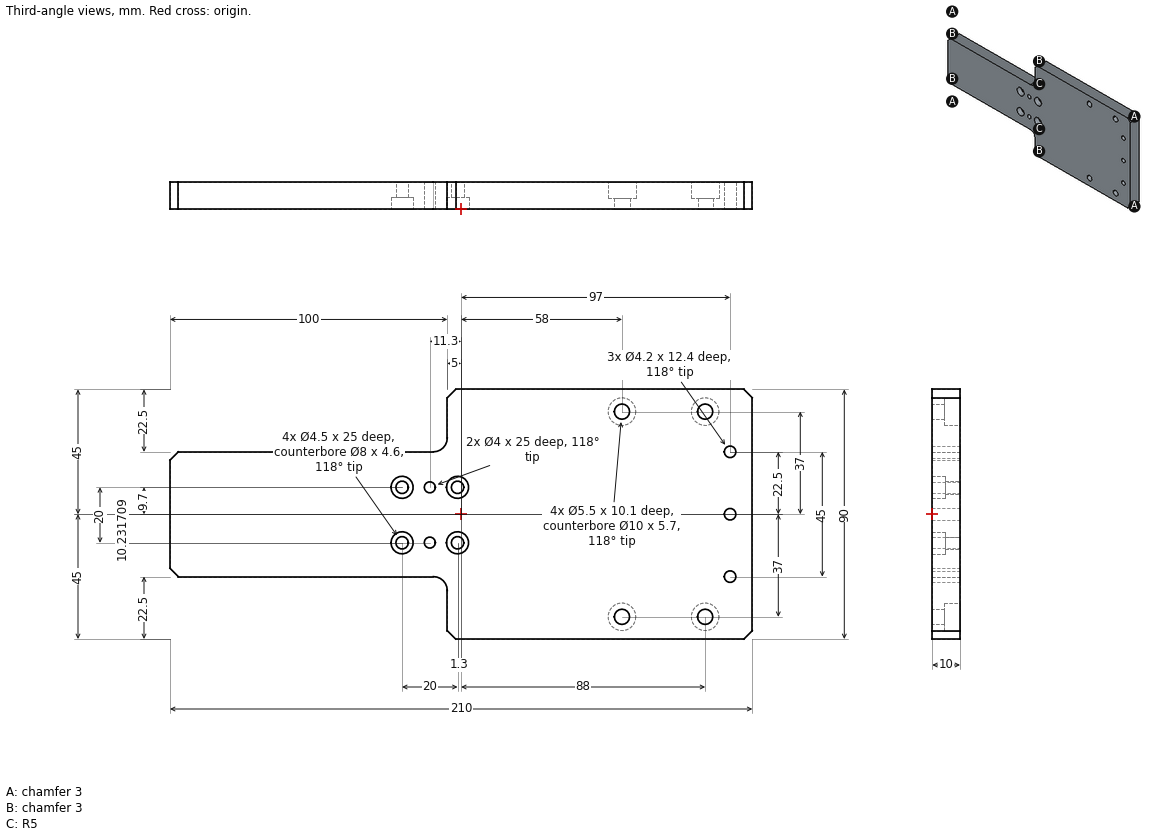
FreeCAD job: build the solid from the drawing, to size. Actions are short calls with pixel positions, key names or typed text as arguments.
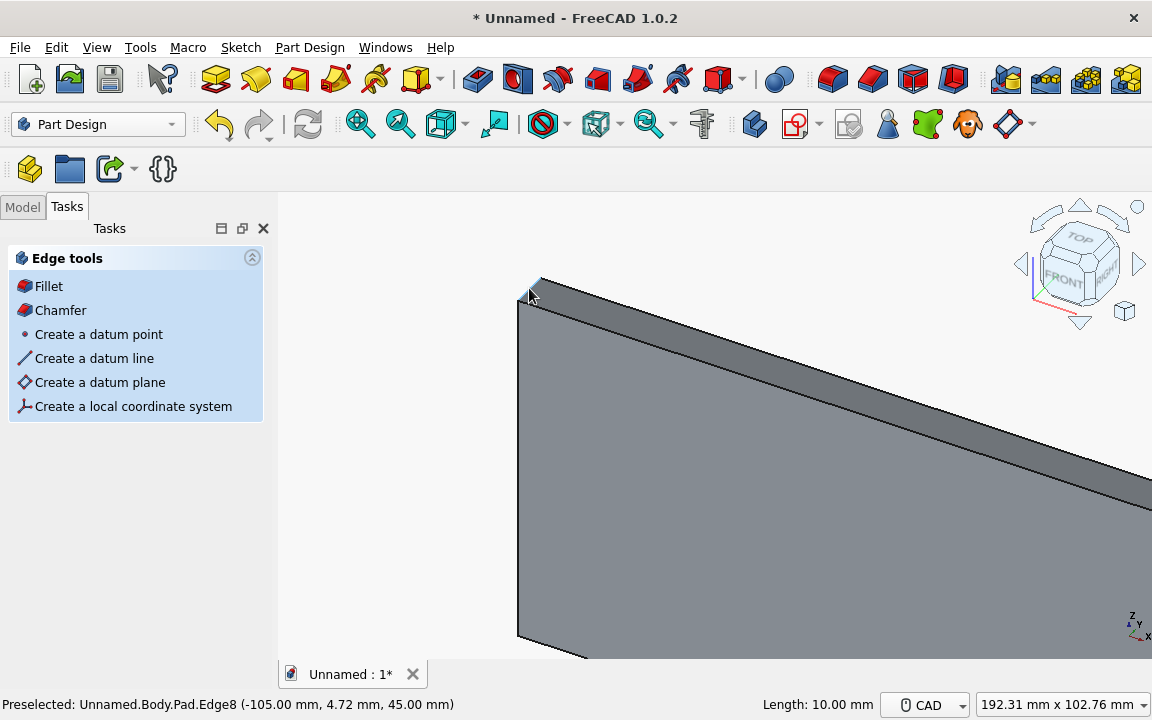
click(362, 124)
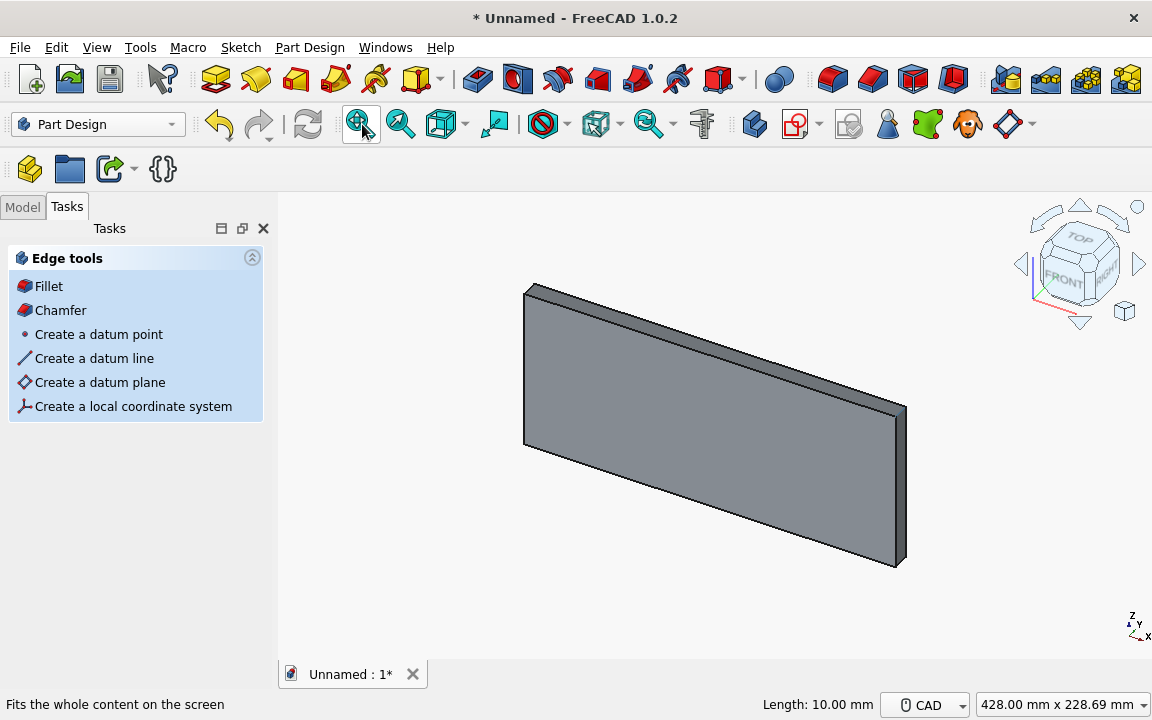
key(0)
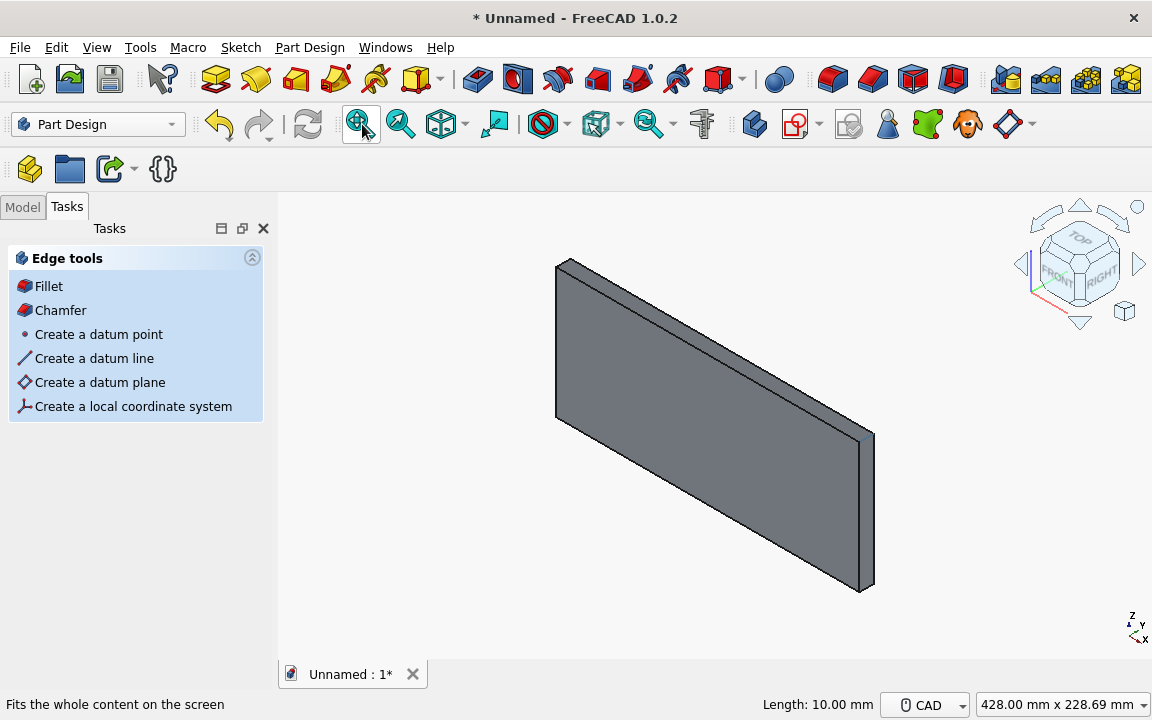
scroll(563, 262, up, 4)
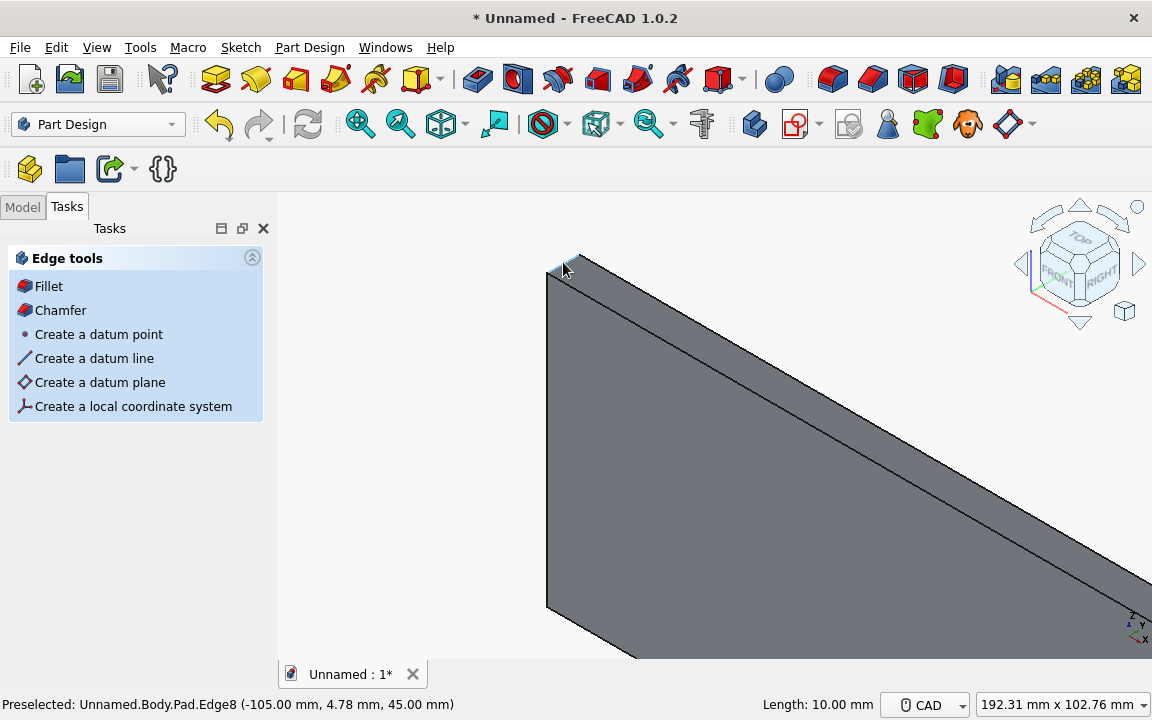
click(362, 124)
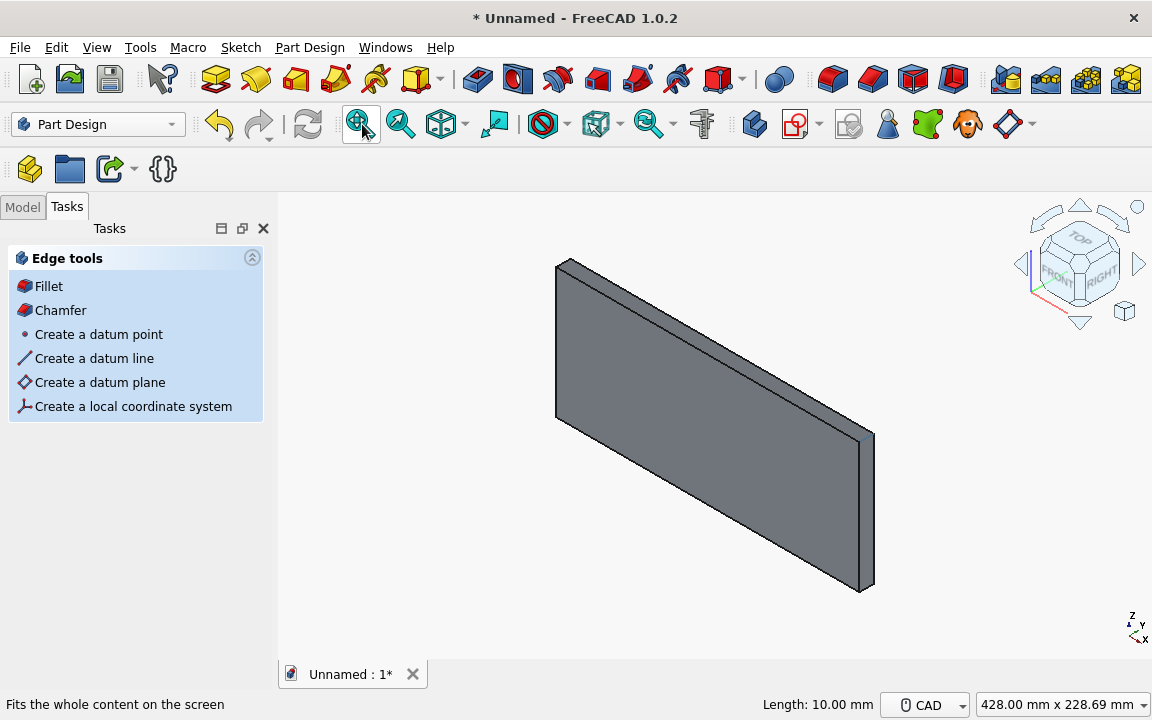
key(2)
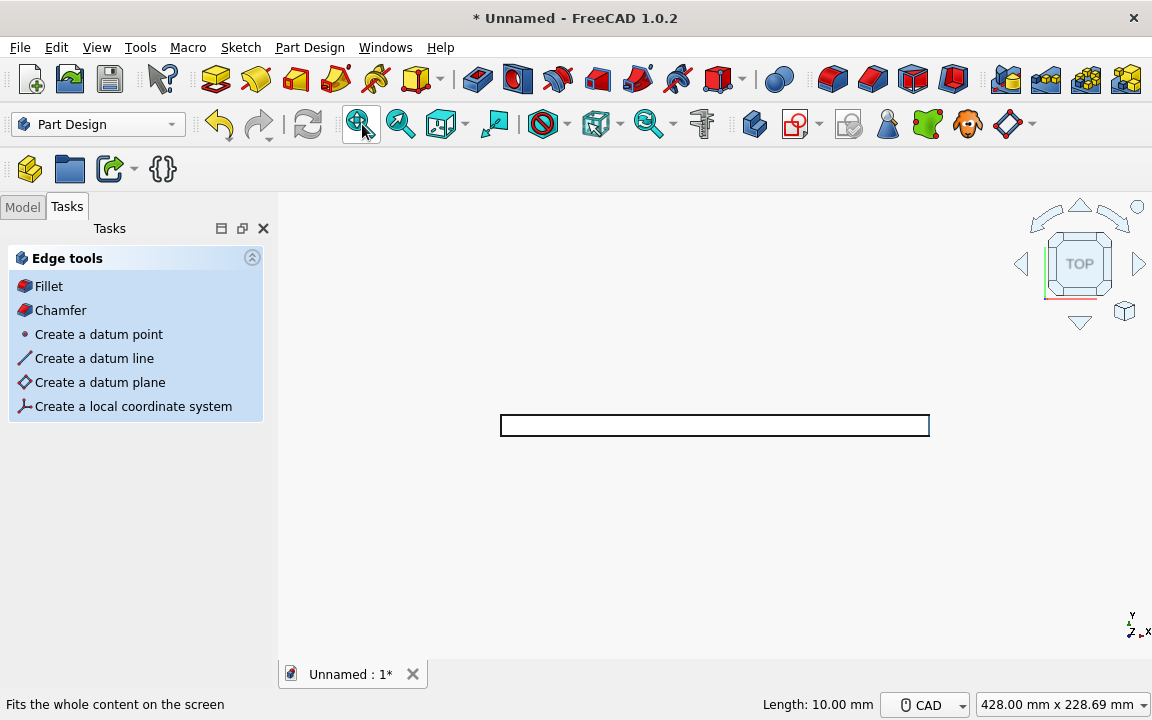
click(501, 424, ctrl)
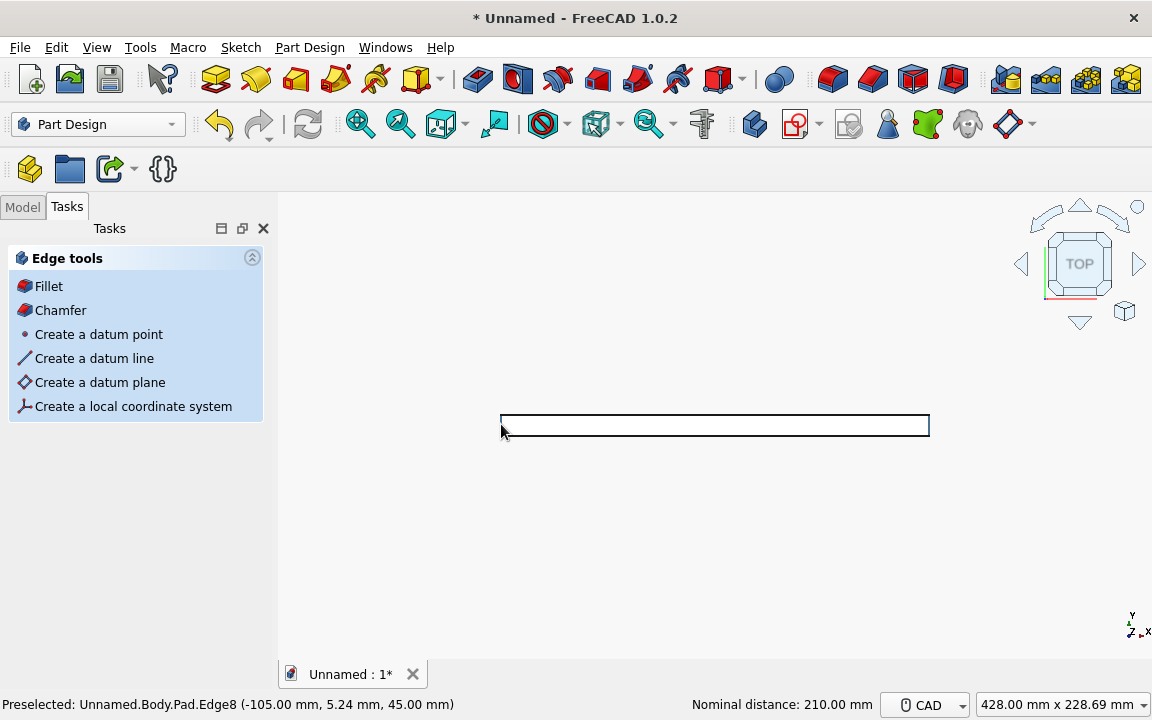
scroll(501, 424, up, 4)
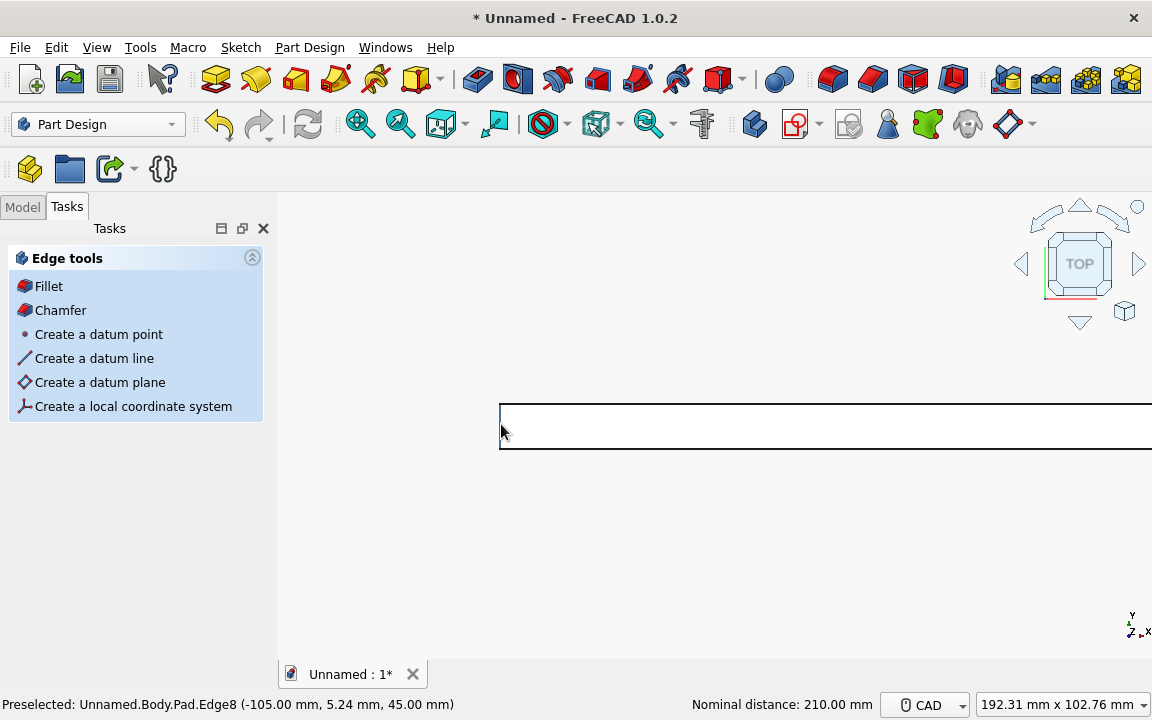
click(362, 124)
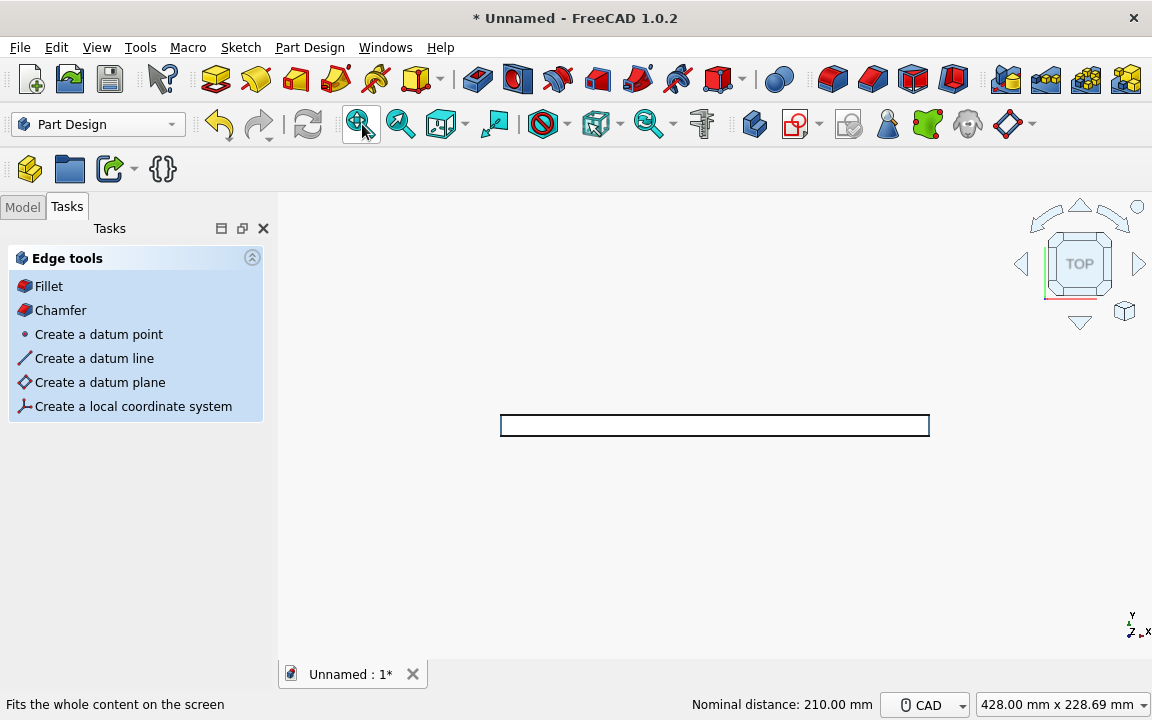
key(1)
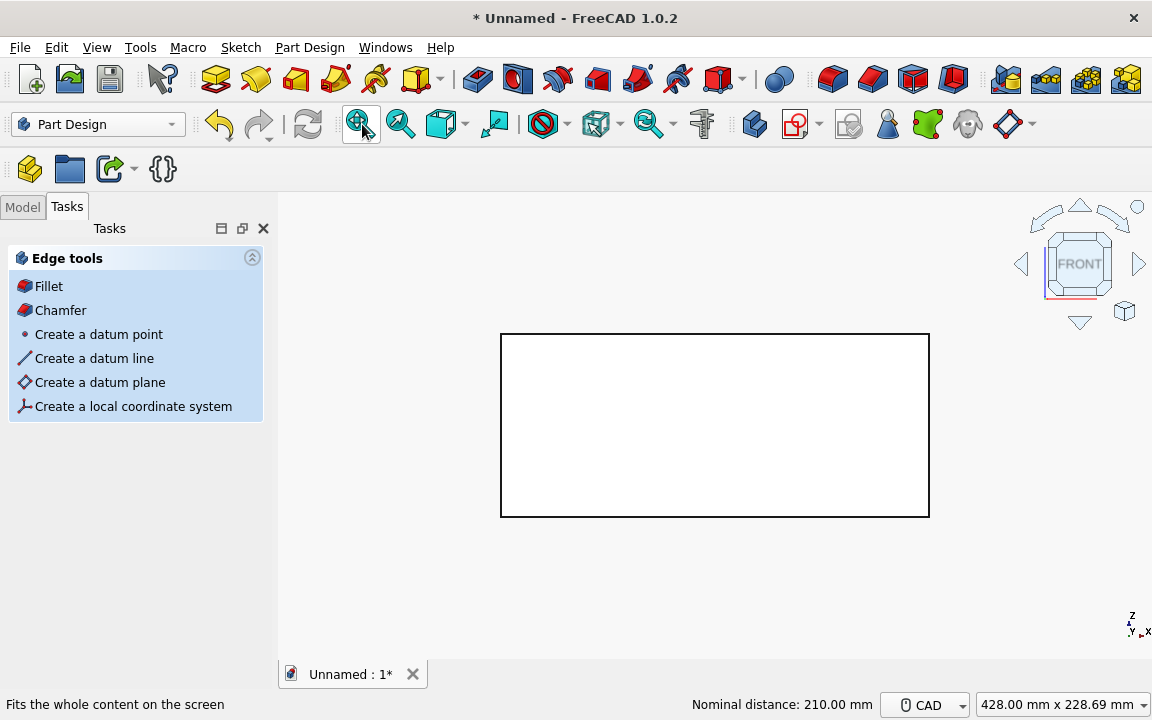
scroll(501, 516, up, 4)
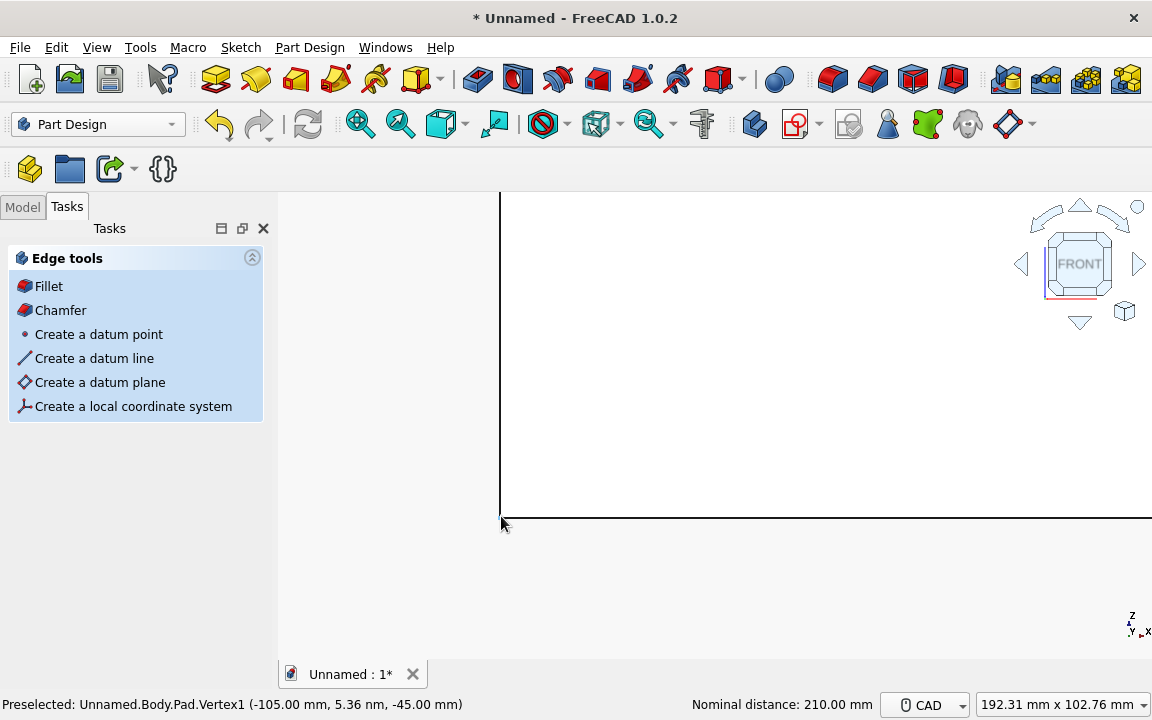
click(362, 124)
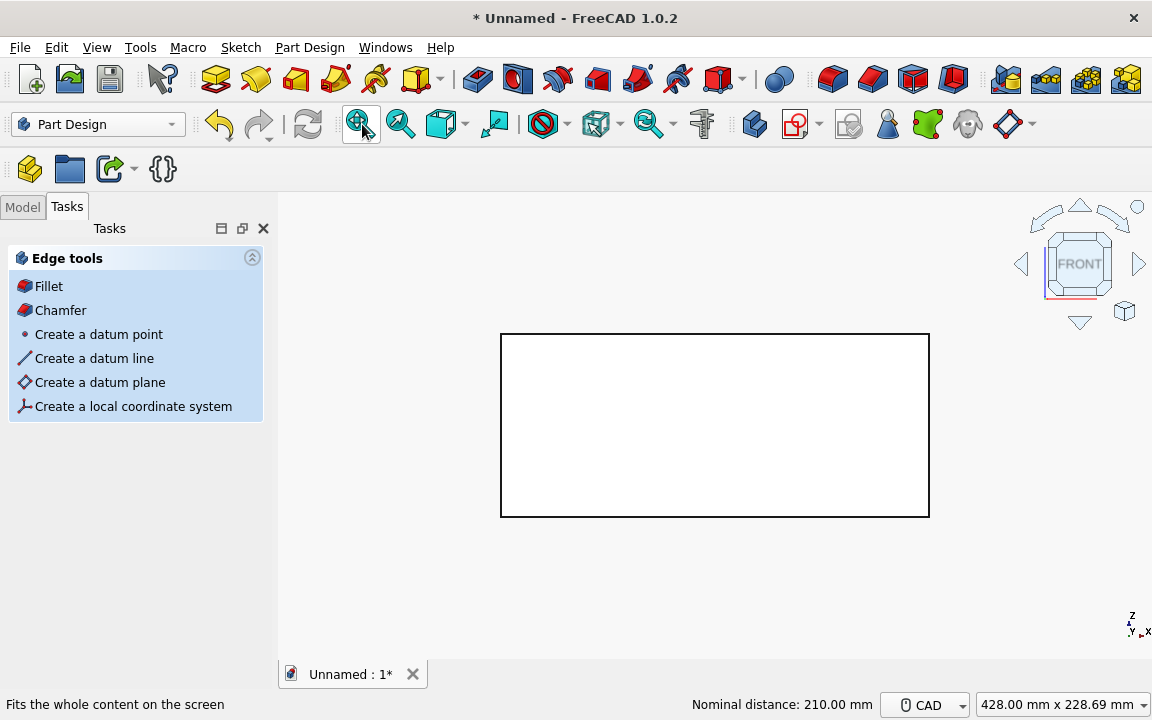
key(3)